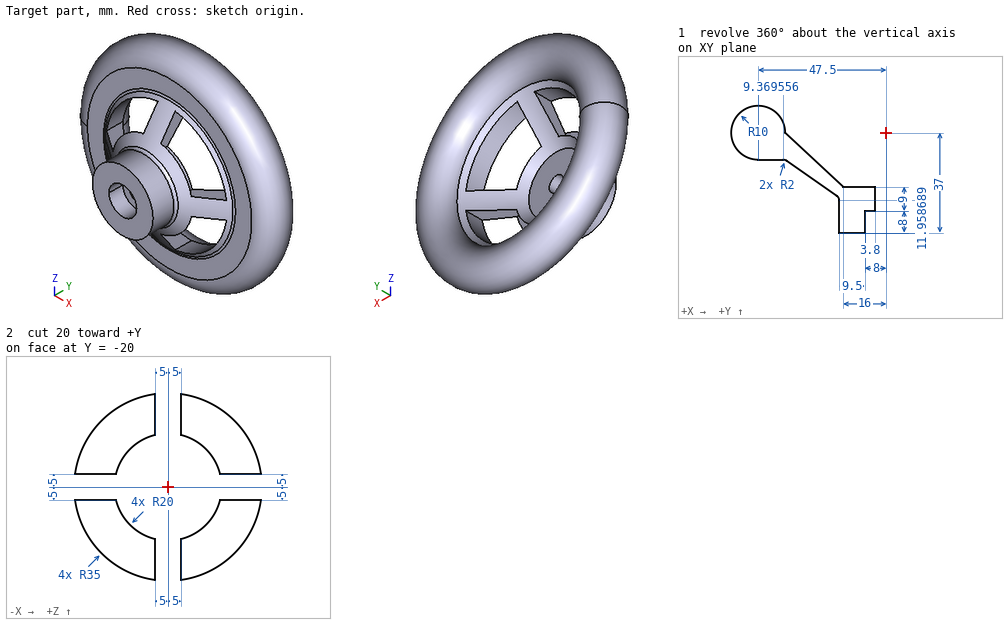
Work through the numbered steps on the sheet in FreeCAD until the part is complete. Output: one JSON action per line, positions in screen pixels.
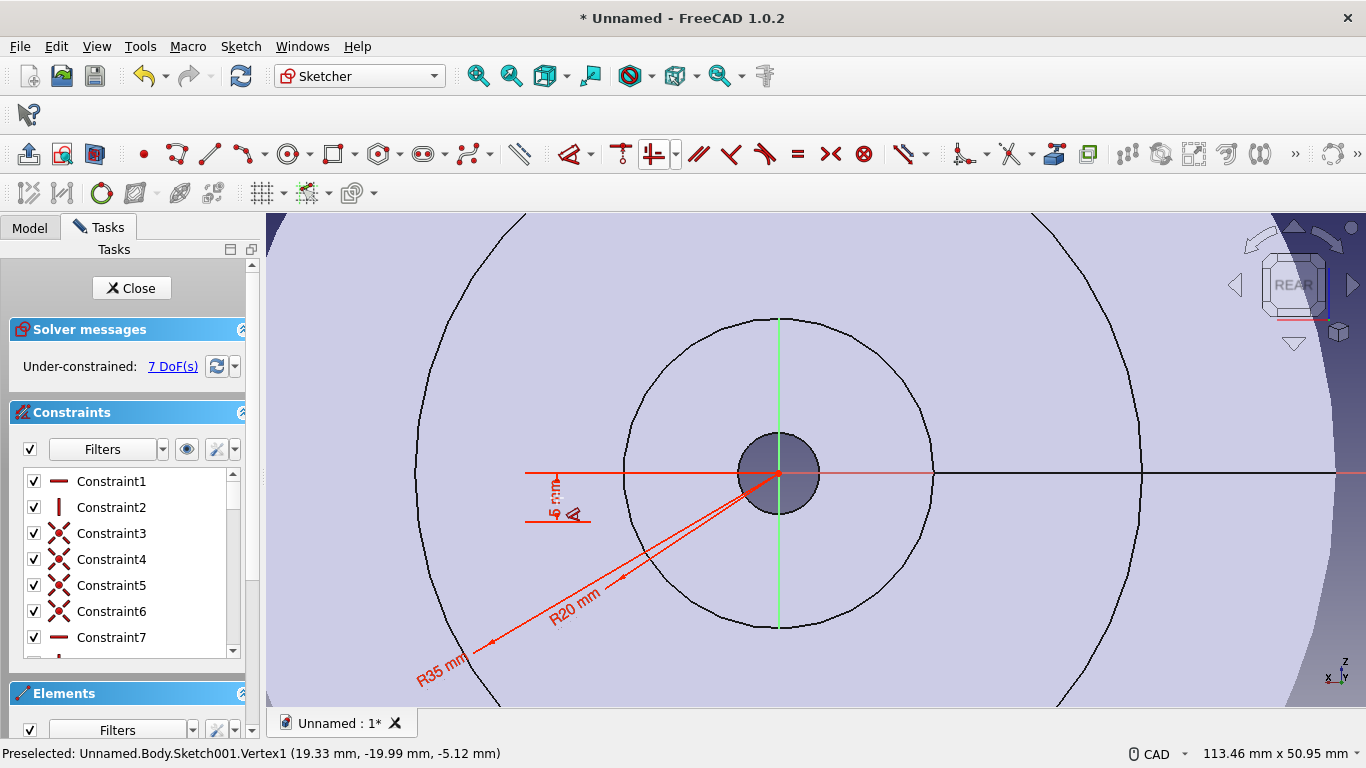
{"action": "scroll", "coordinate": [722, 449], "scroll_direction": "down", "scroll_amount": 4}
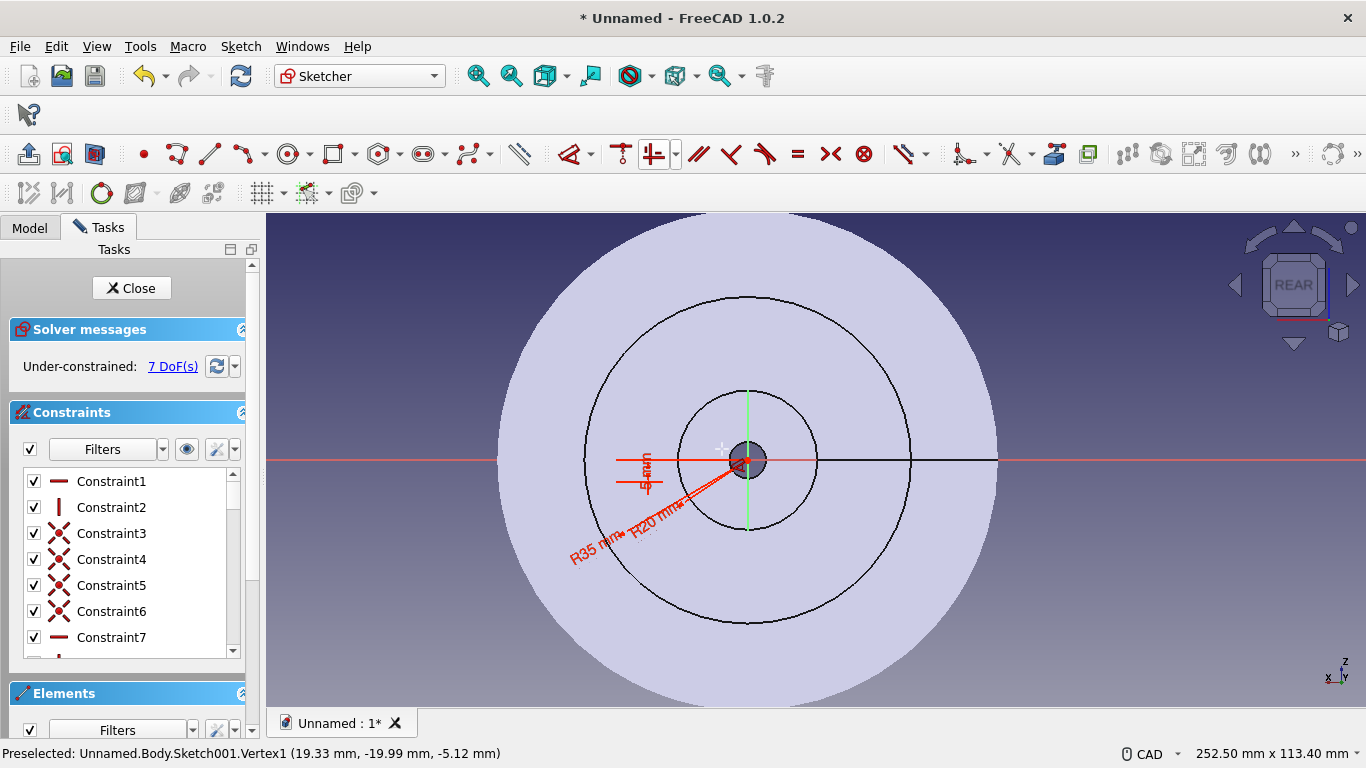
{"action": "scroll", "coordinate": [726, 611], "scroll_direction": "up", "scroll_amount": 4}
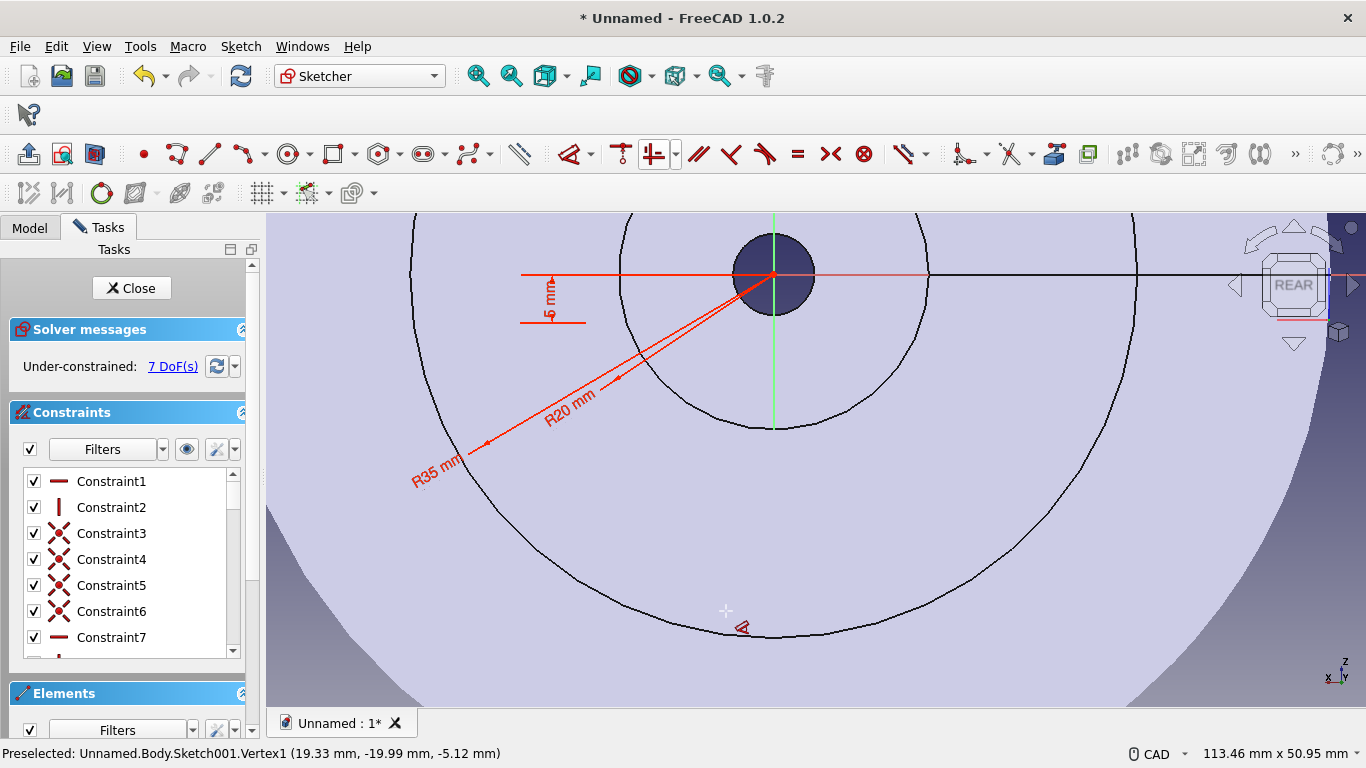
{"action": "left_click", "coordinate": [726, 611]}
{"action": "left_click", "coordinate": [750, 645]}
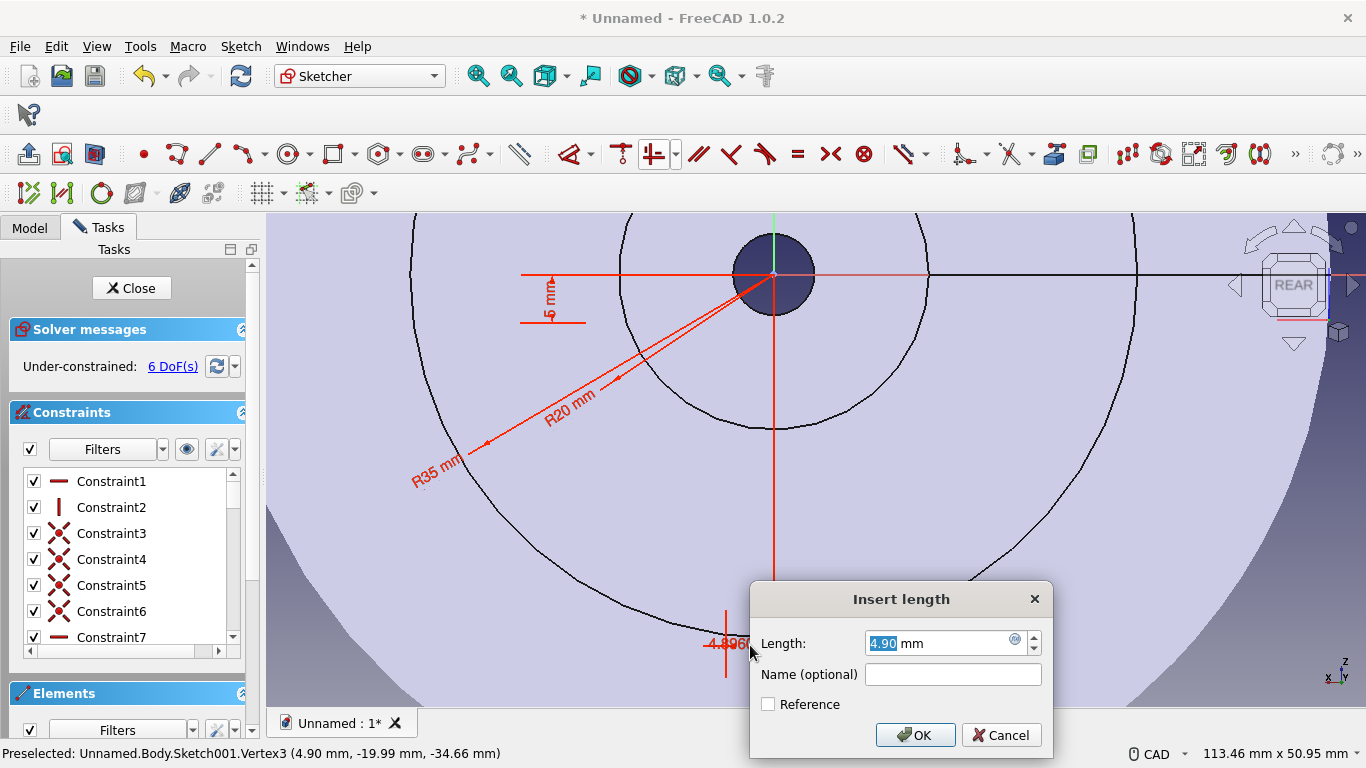
{"action": "type", "text": "5"}
{"action": "key", "text": "Return"}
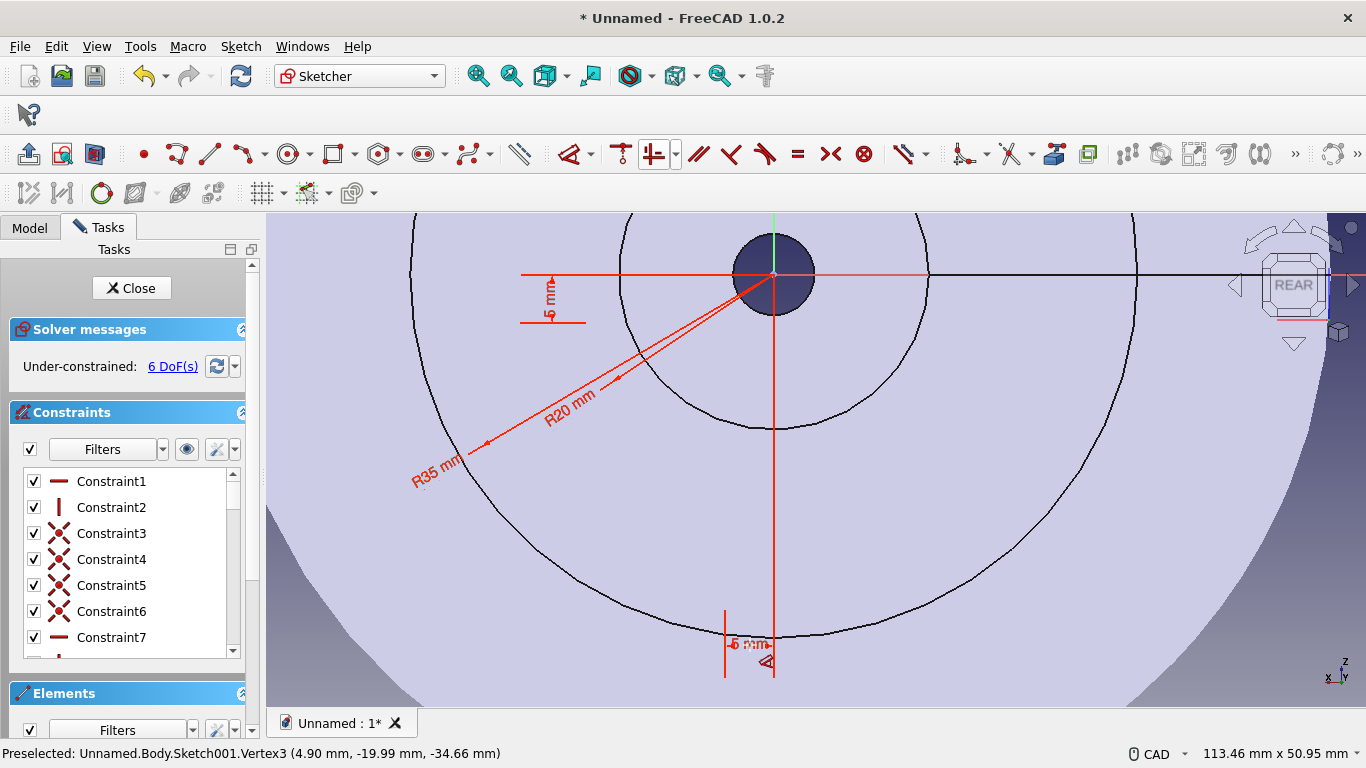
{"action": "scroll", "coordinate": [726, 611], "scroll_direction": "down", "scroll_amount": 4}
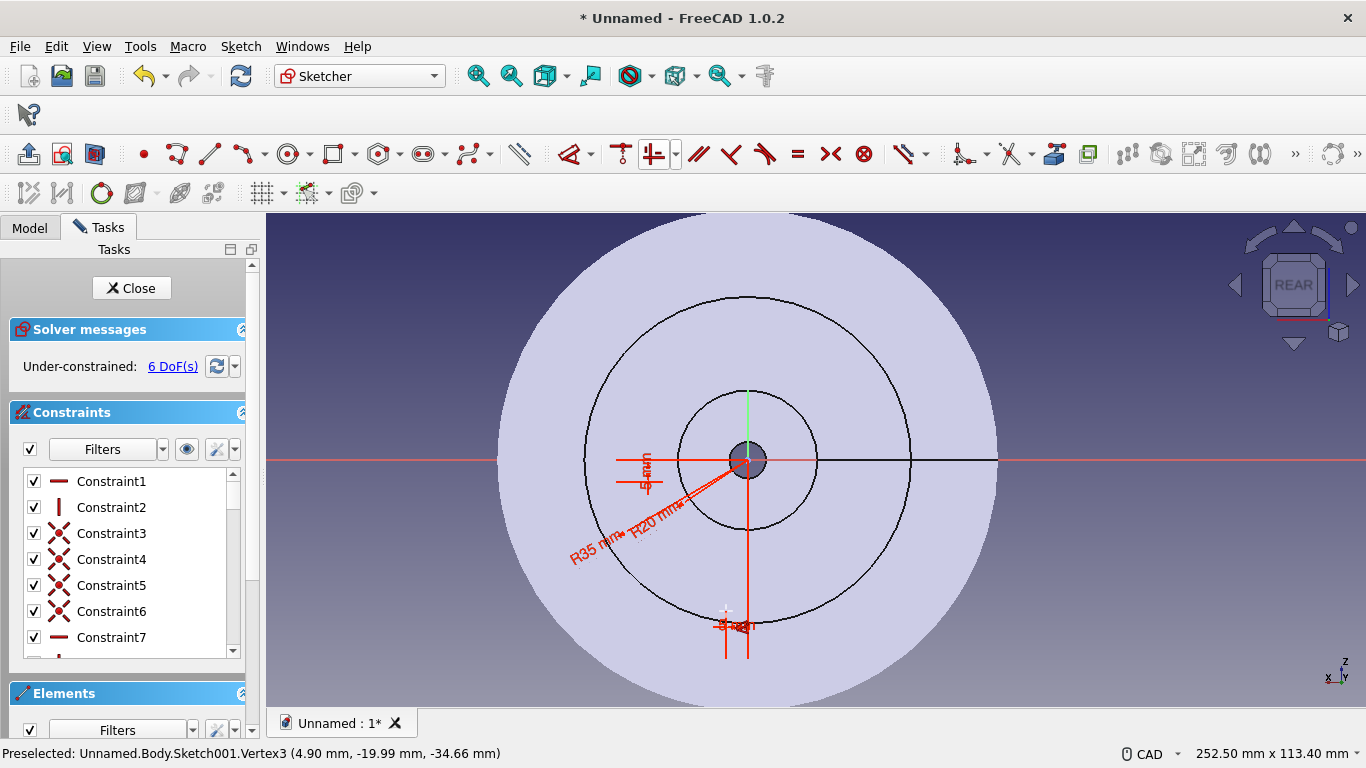
{"action": "scroll", "coordinate": [597, 439], "scroll_direction": "up", "scroll_amount": 4}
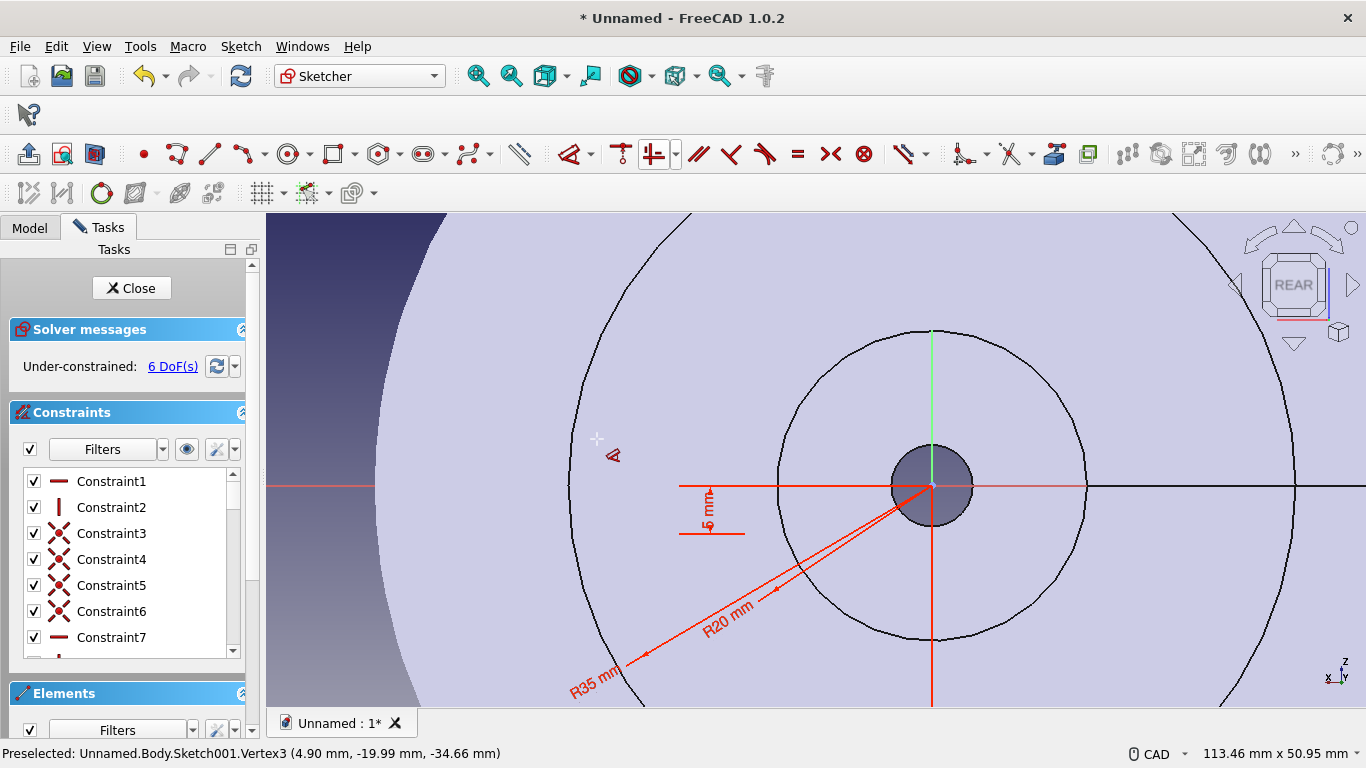
{"action": "left_click", "coordinate": [596, 439]}
{"action": "left_click", "coordinate": [562, 462]}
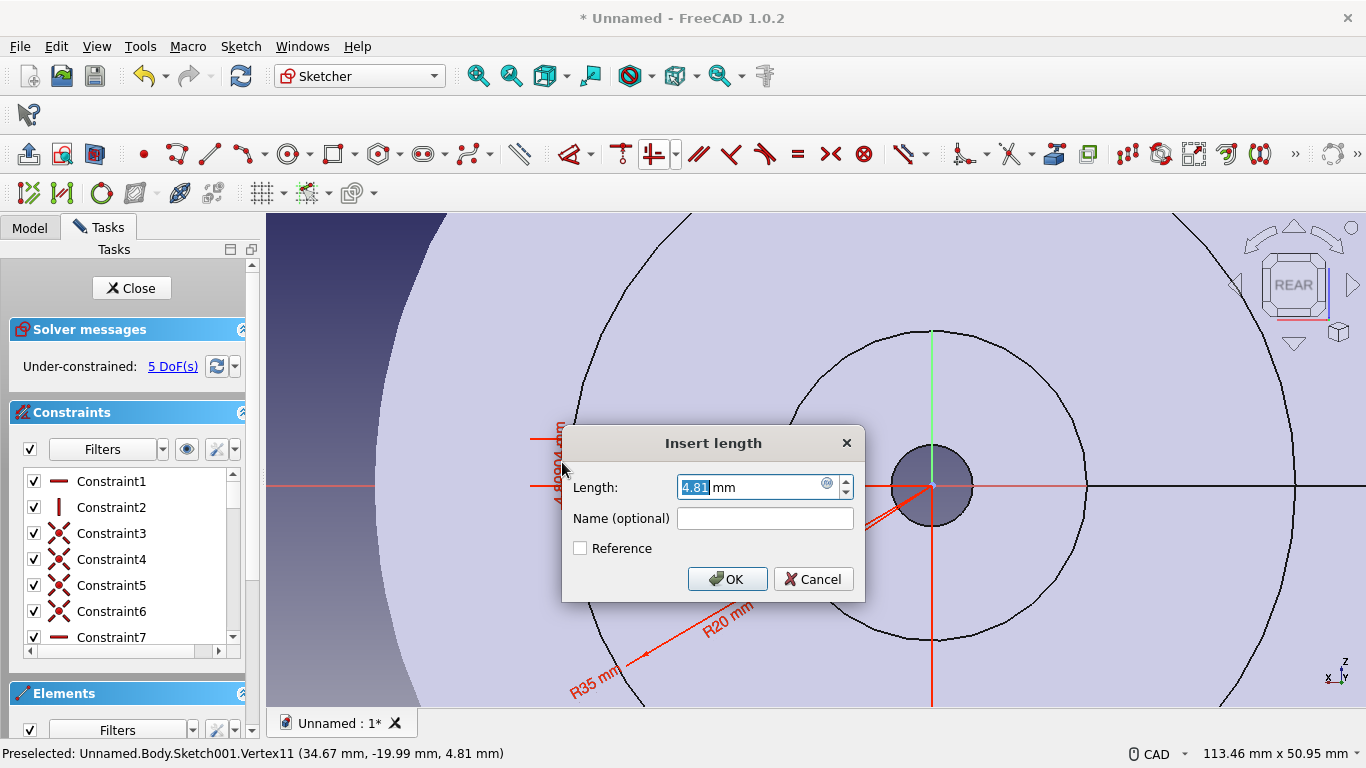
{"action": "type", "text": "5"}
{"action": "key", "text": "Return"}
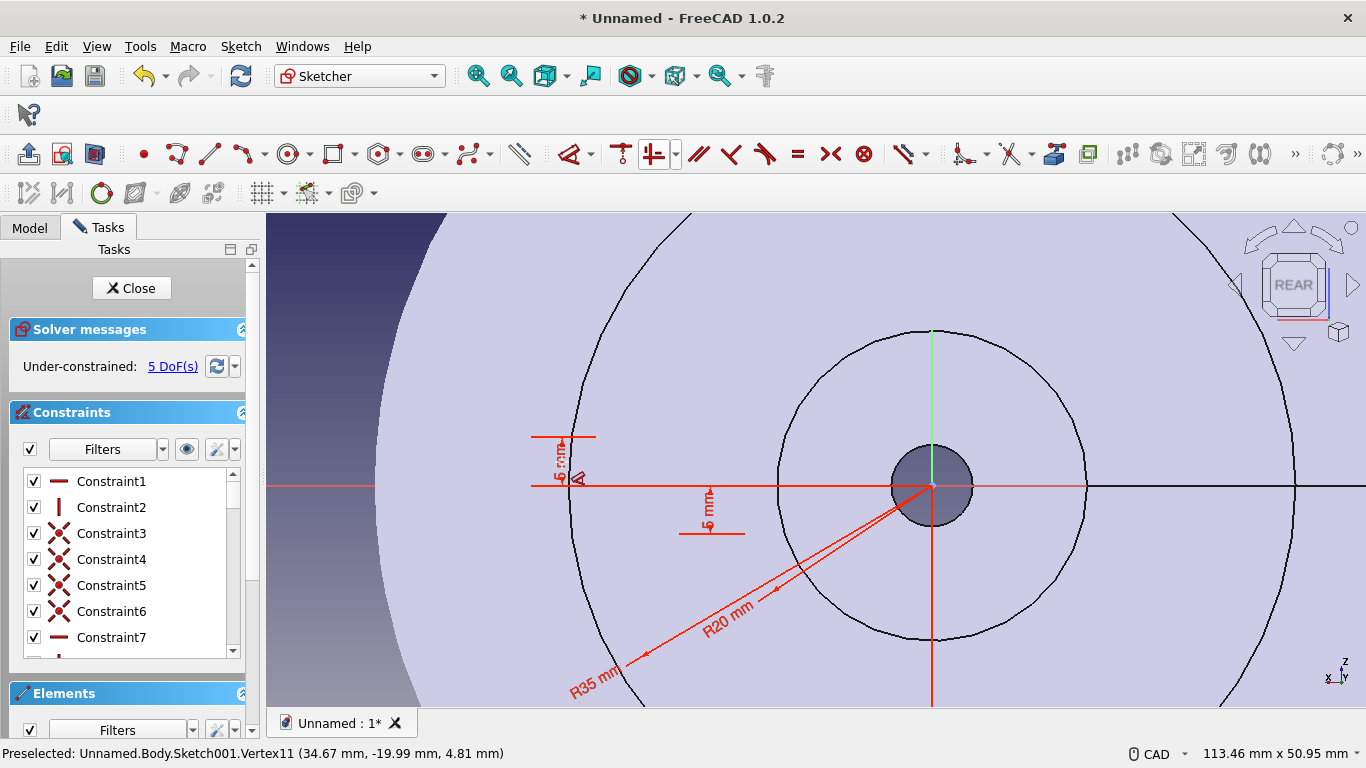
{"action": "left_click", "coordinate": [884, 298]}
{"action": "left_click", "coordinate": [908, 264]}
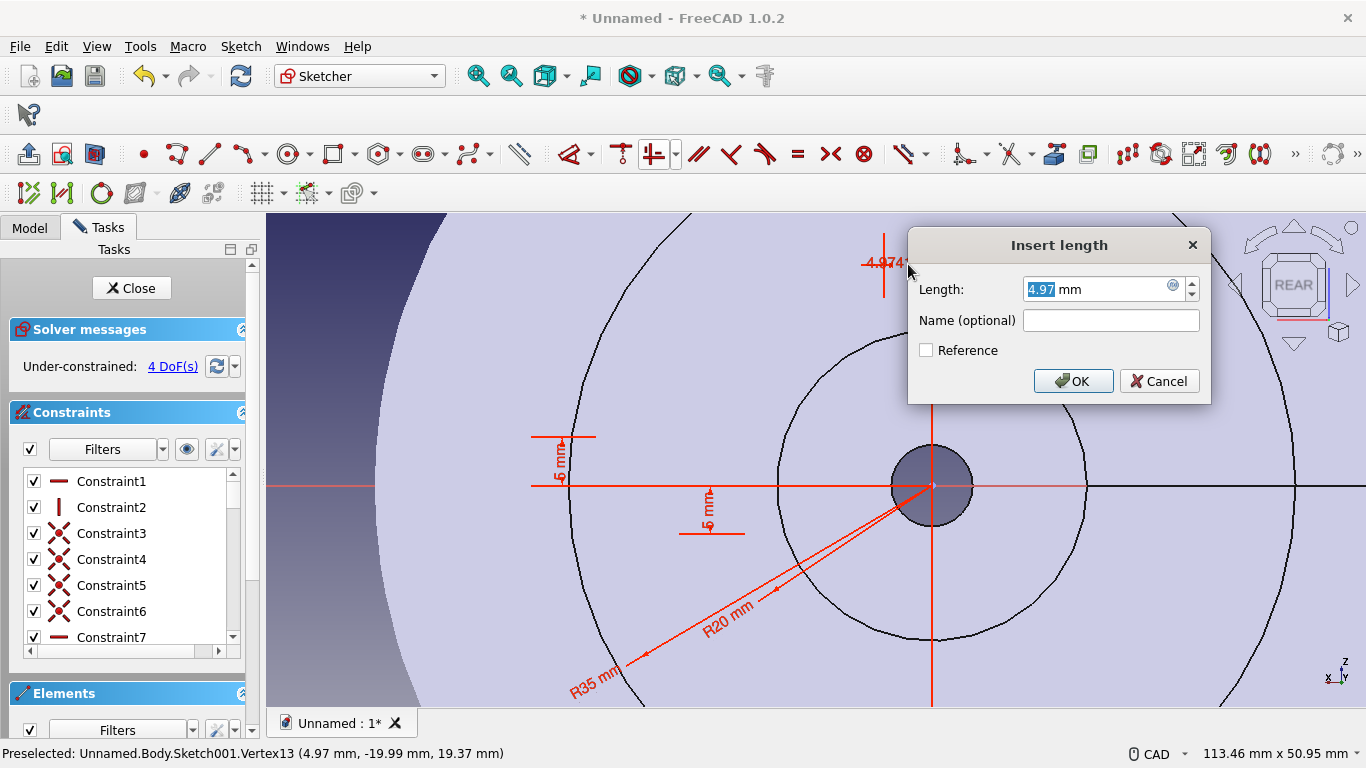
{"action": "type", "text": "5"}
{"action": "key", "text": "Return"}